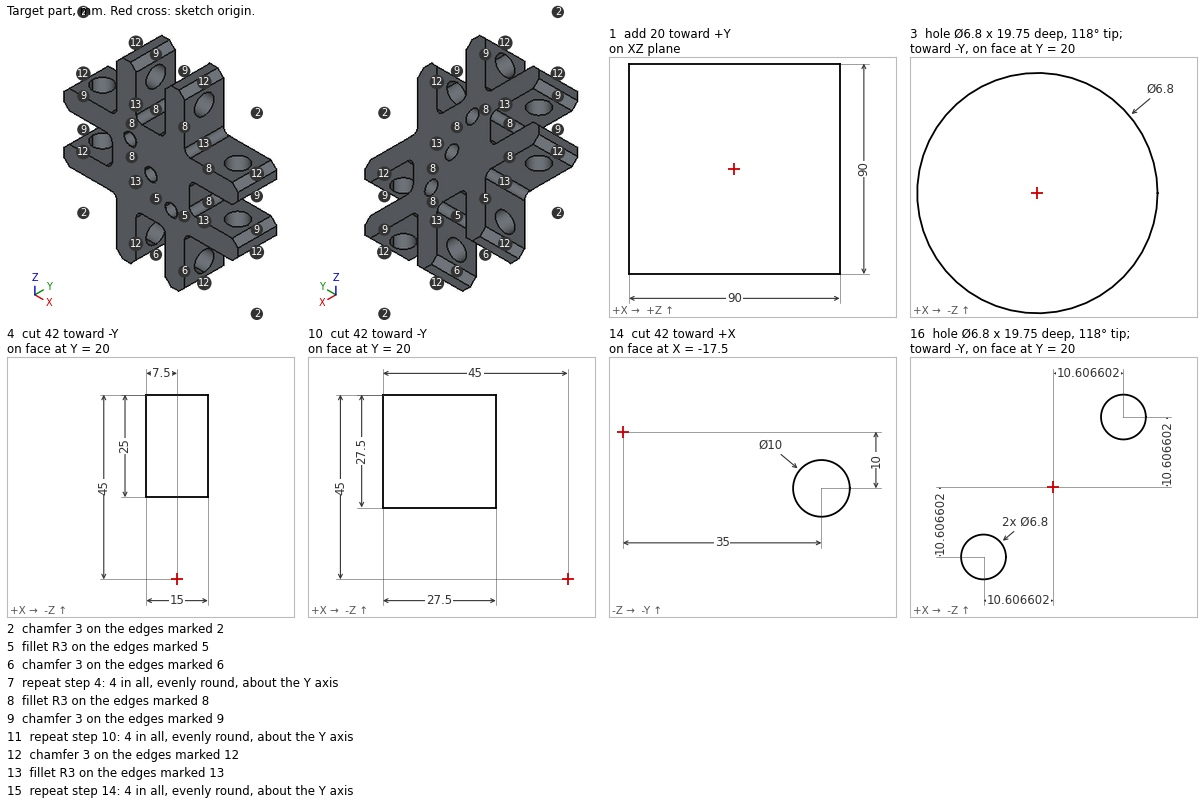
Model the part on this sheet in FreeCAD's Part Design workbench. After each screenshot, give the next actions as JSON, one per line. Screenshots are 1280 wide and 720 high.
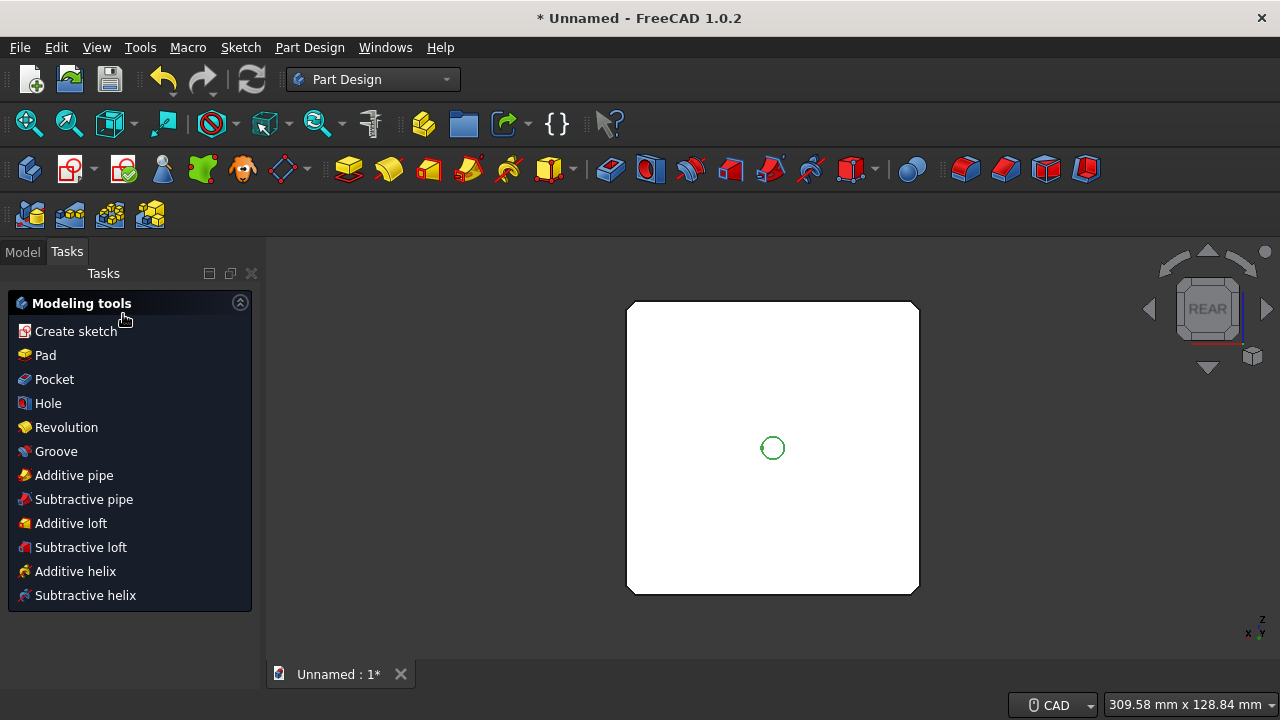
{"action": "left_click", "coordinate": [652, 170]}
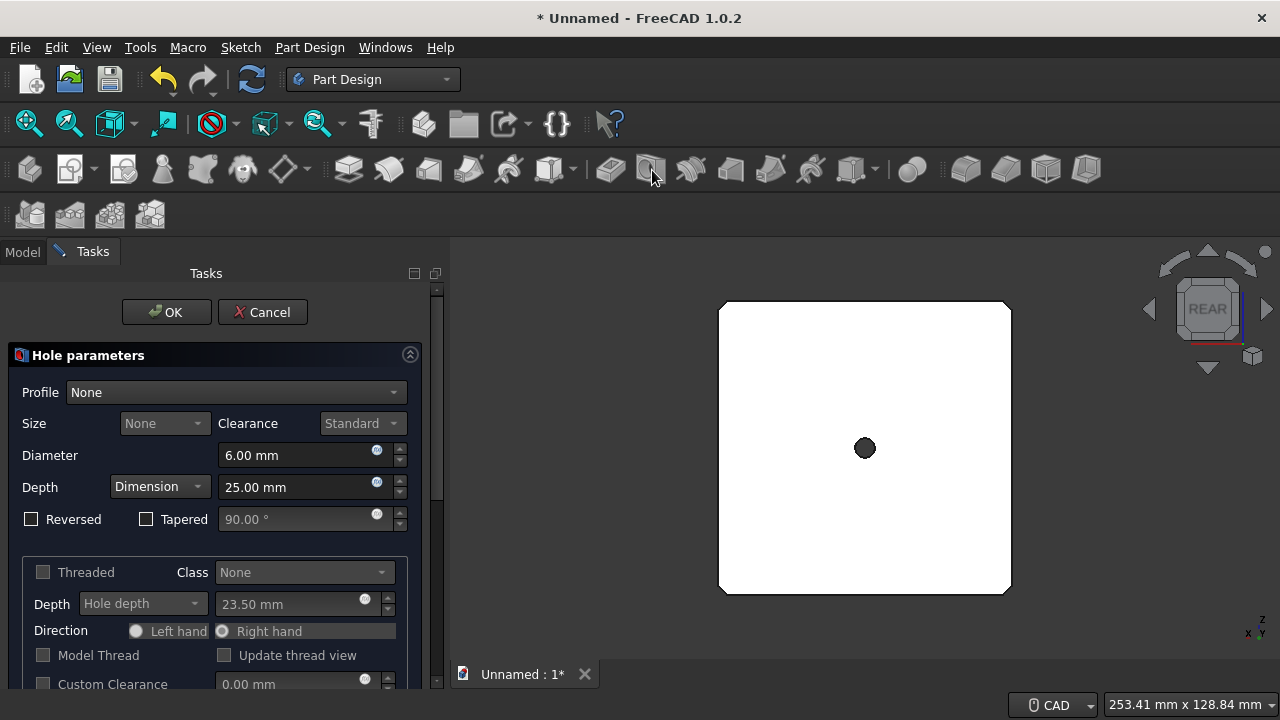
{"action": "triple_click", "coordinate": [305, 455]}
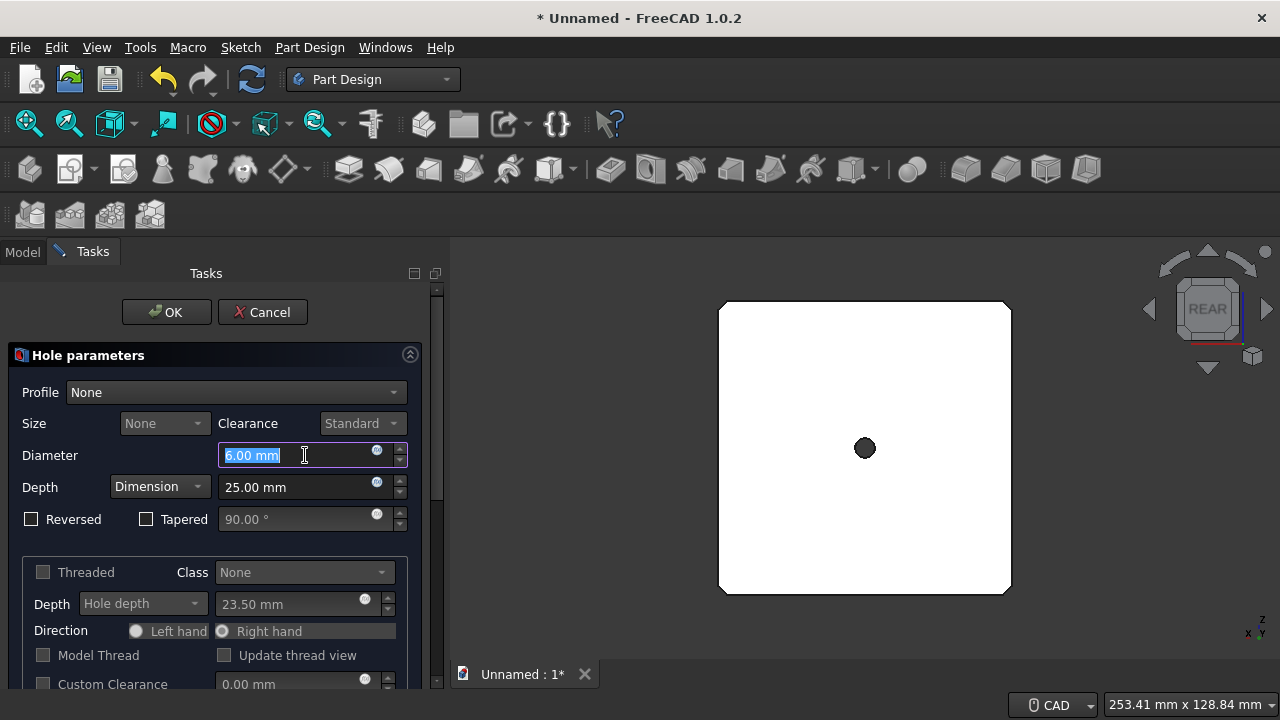
{"action": "type", "text": "6.8"}
{"action": "key", "text": "Tab"}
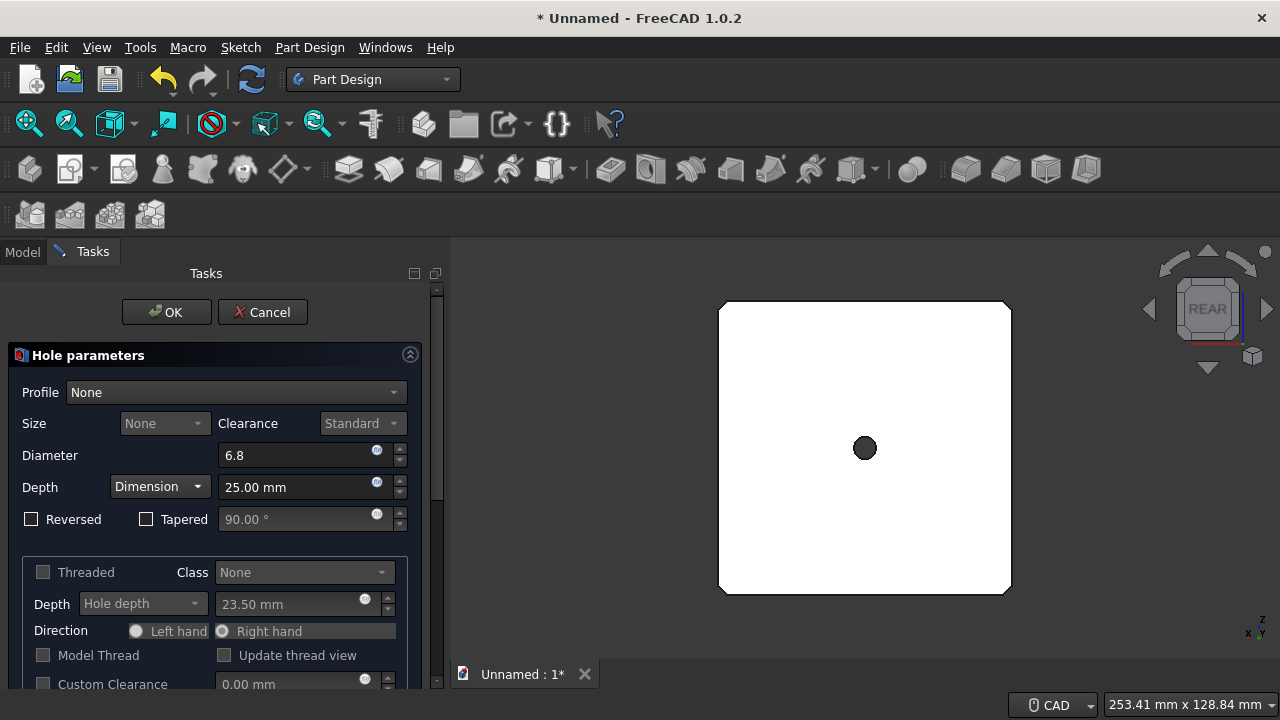
{"action": "triple_click", "coordinate": [305, 487]}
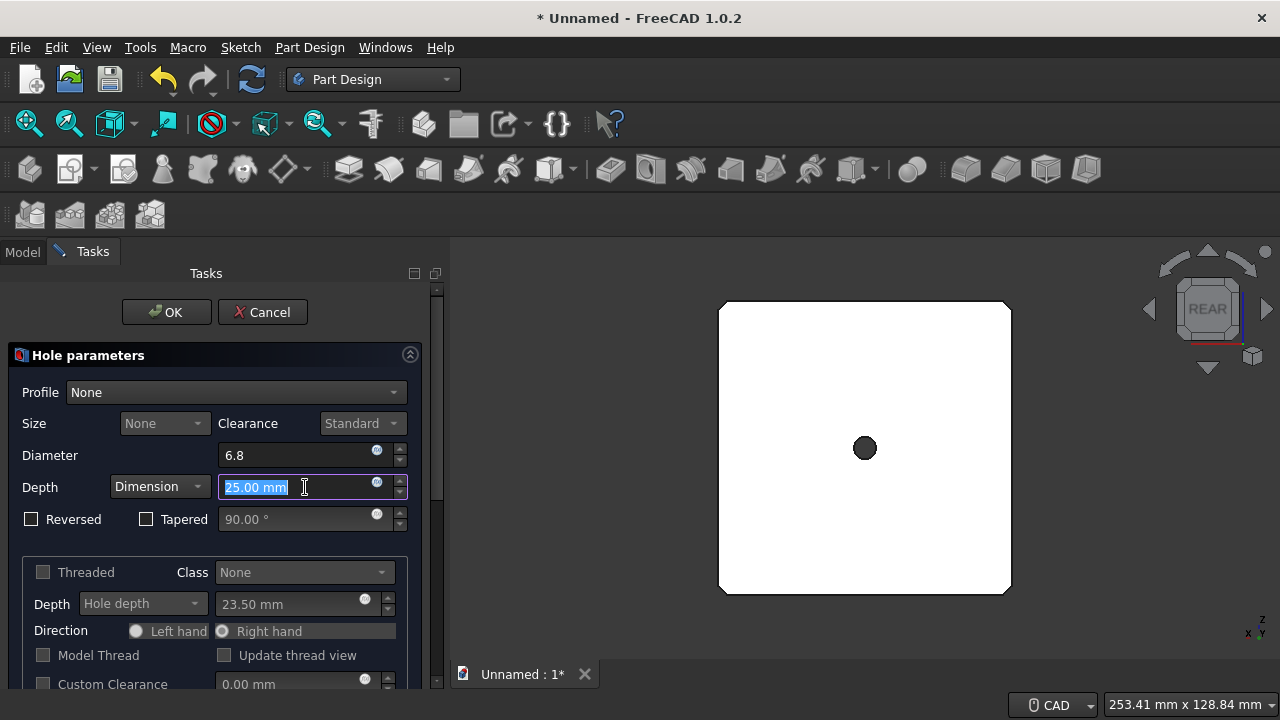
{"action": "type", "text": "19.75"}
{"action": "key", "text": "Tab"}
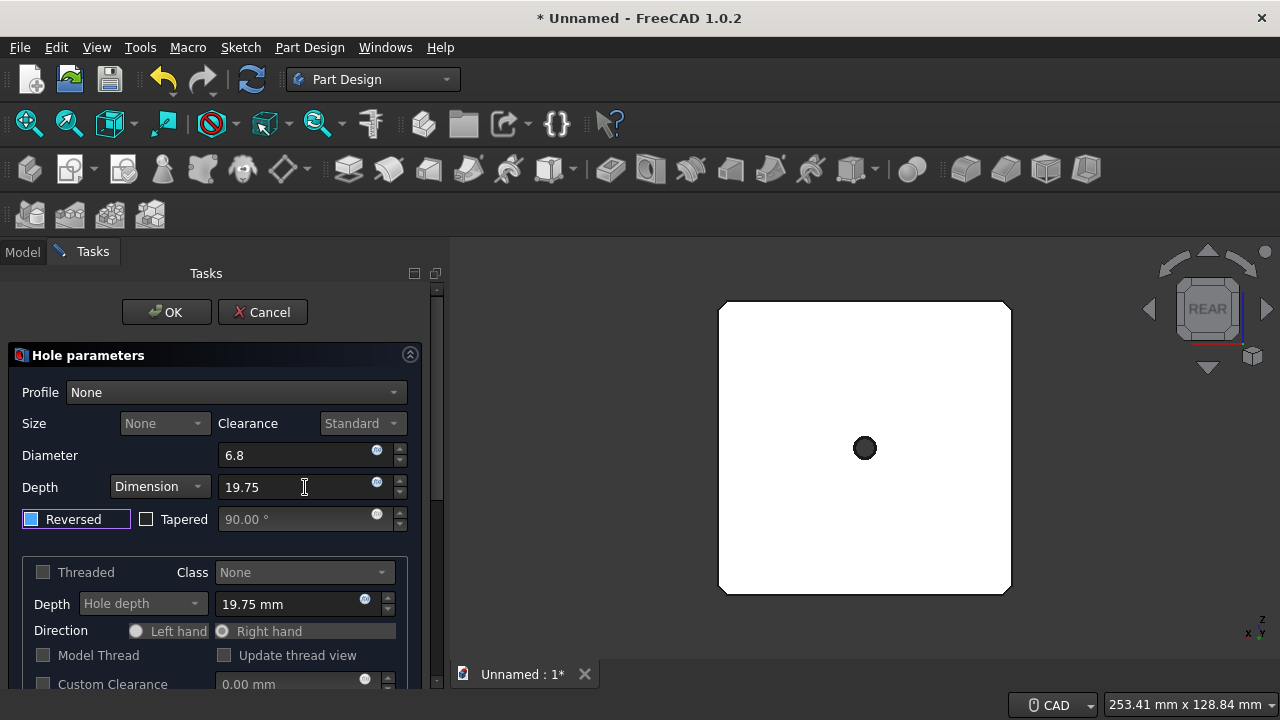
{"action": "left_click", "coordinate": [167, 312]}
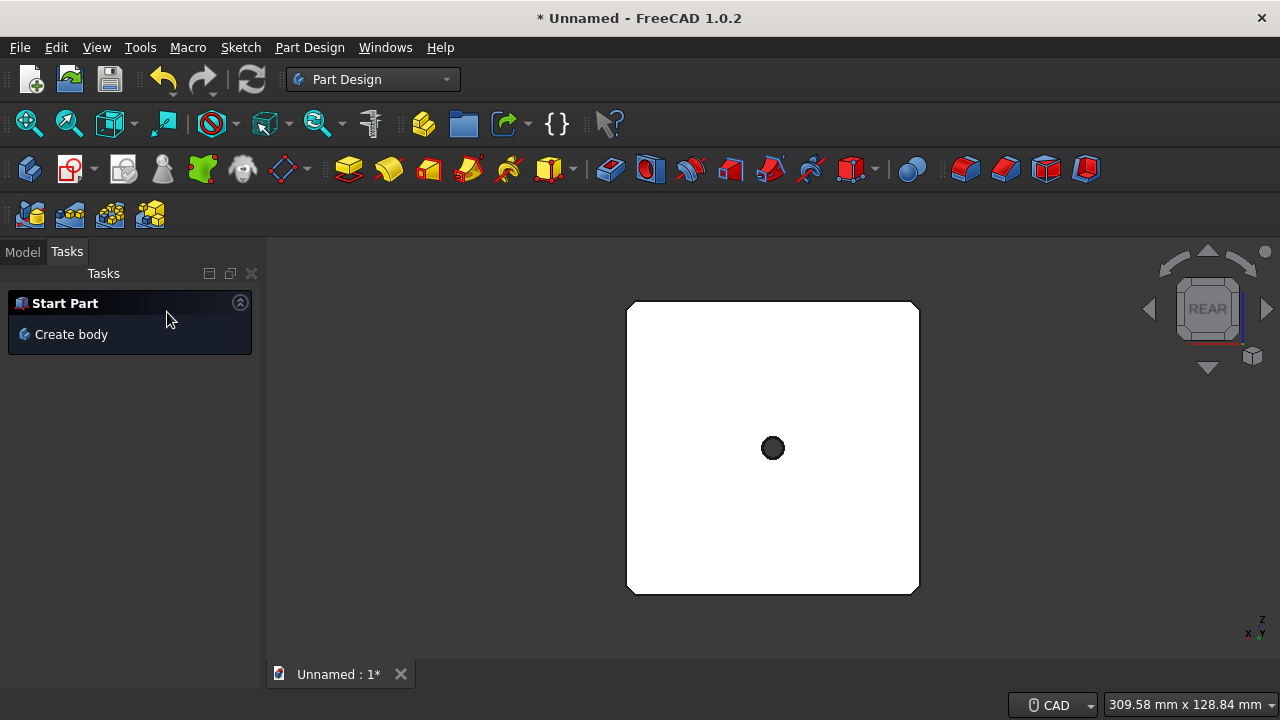
{"action": "left_click", "coordinate": [689, 405]}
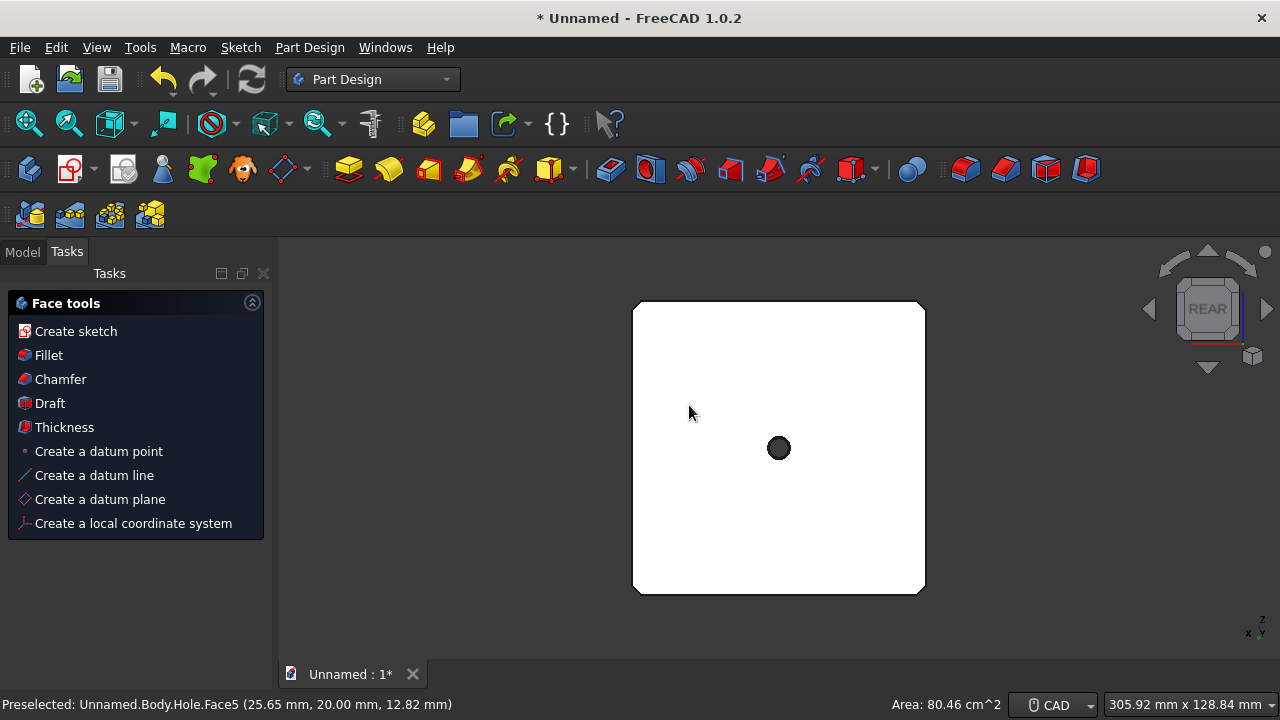
{"action": "left_click", "coordinate": [70, 170]}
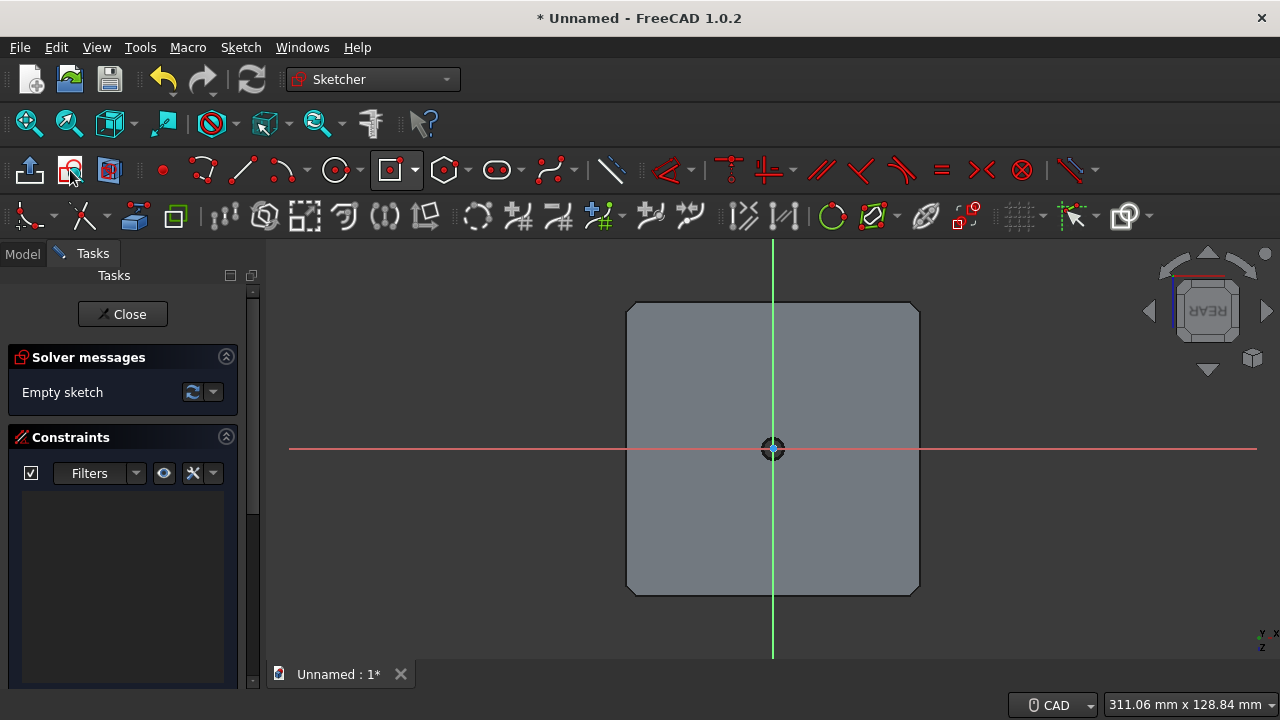
{"action": "scroll", "coordinate": [856, 286], "scroll_direction": "up", "scroll_amount": 3}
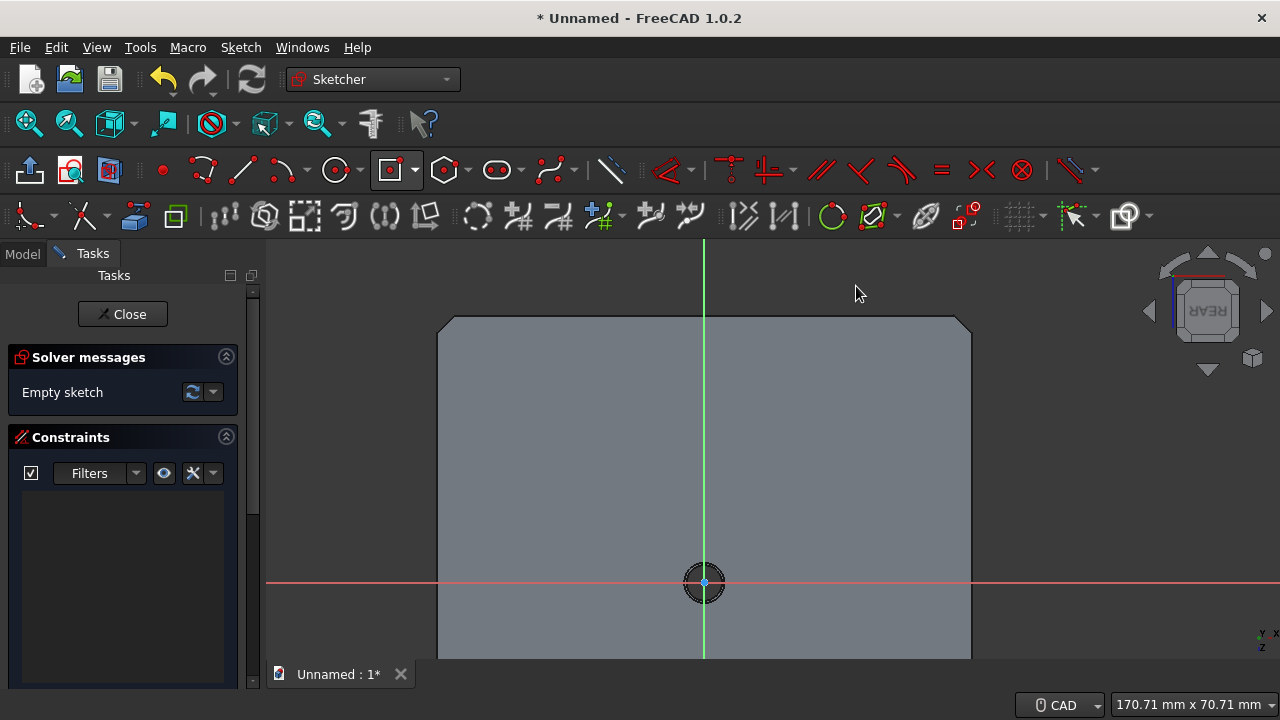
{"action": "key", "text": "g r"}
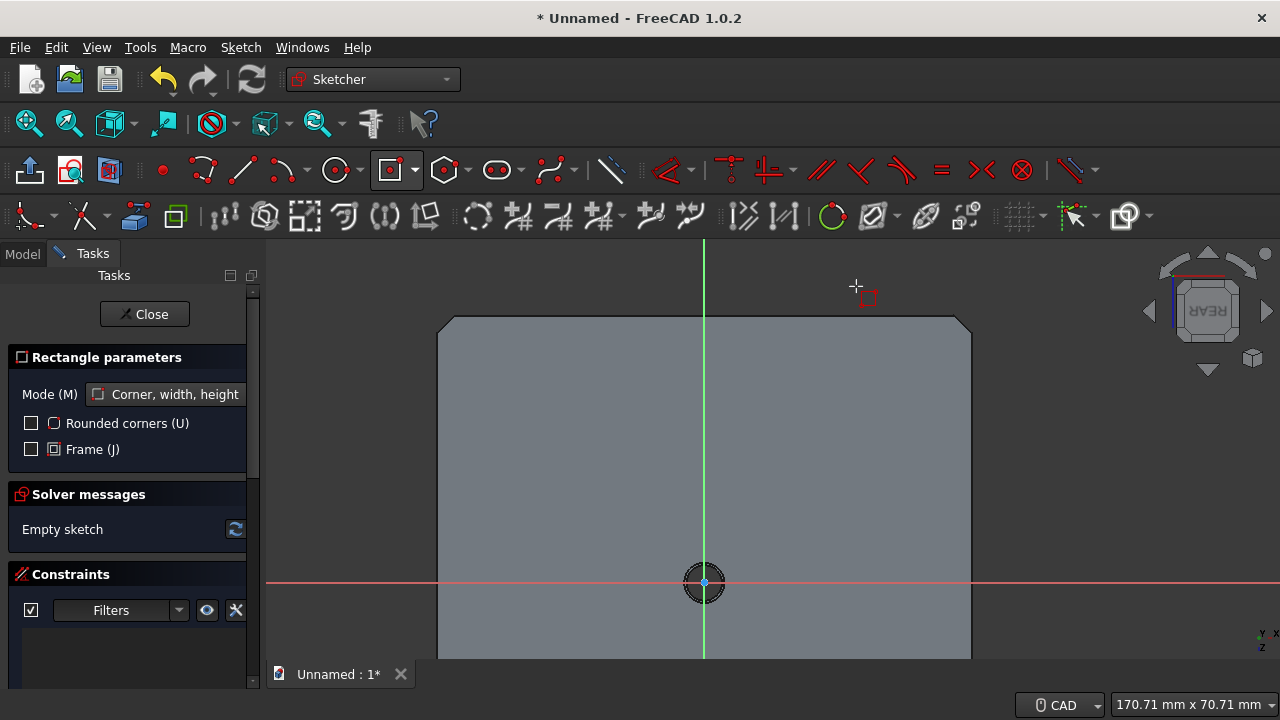
{"action": "left_click", "coordinate": [660, 316]}
{"action": "left_click", "coordinate": [749, 464]}
{"action": "key", "text": "Escape"}